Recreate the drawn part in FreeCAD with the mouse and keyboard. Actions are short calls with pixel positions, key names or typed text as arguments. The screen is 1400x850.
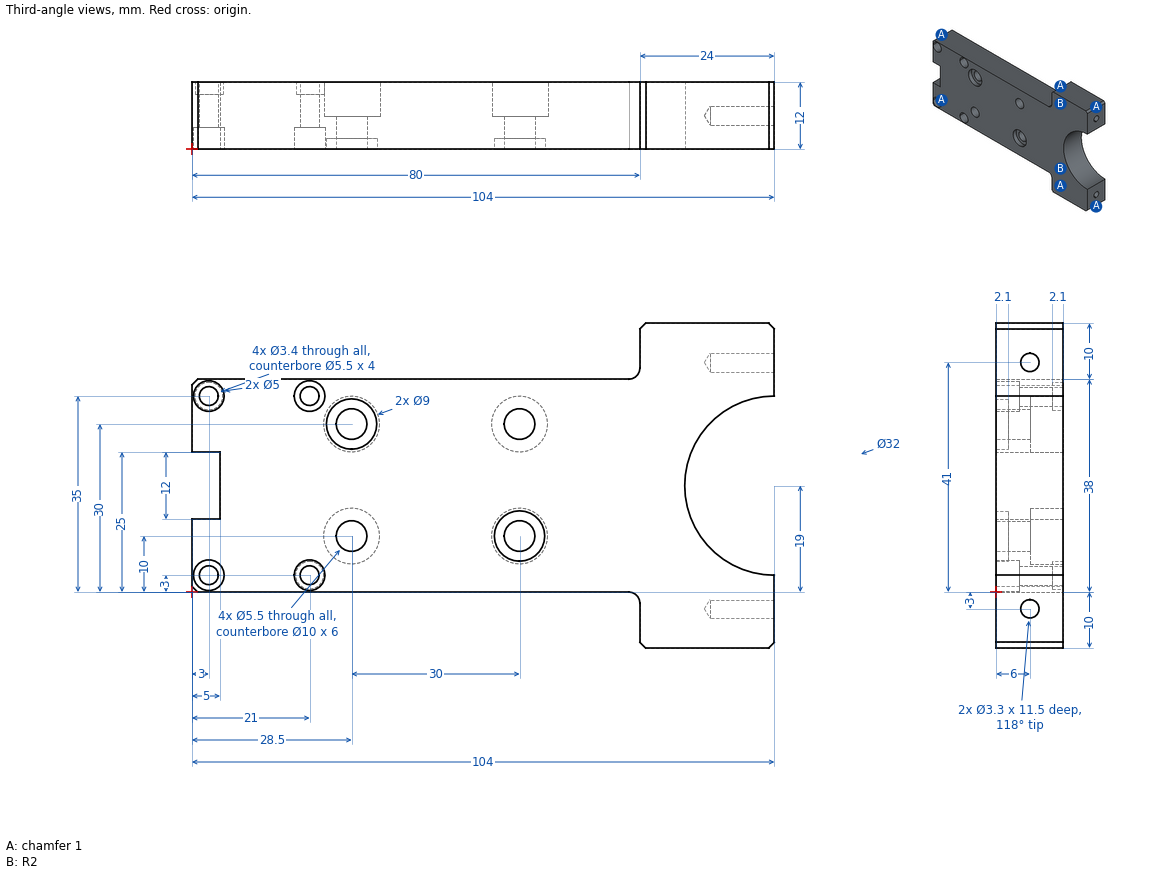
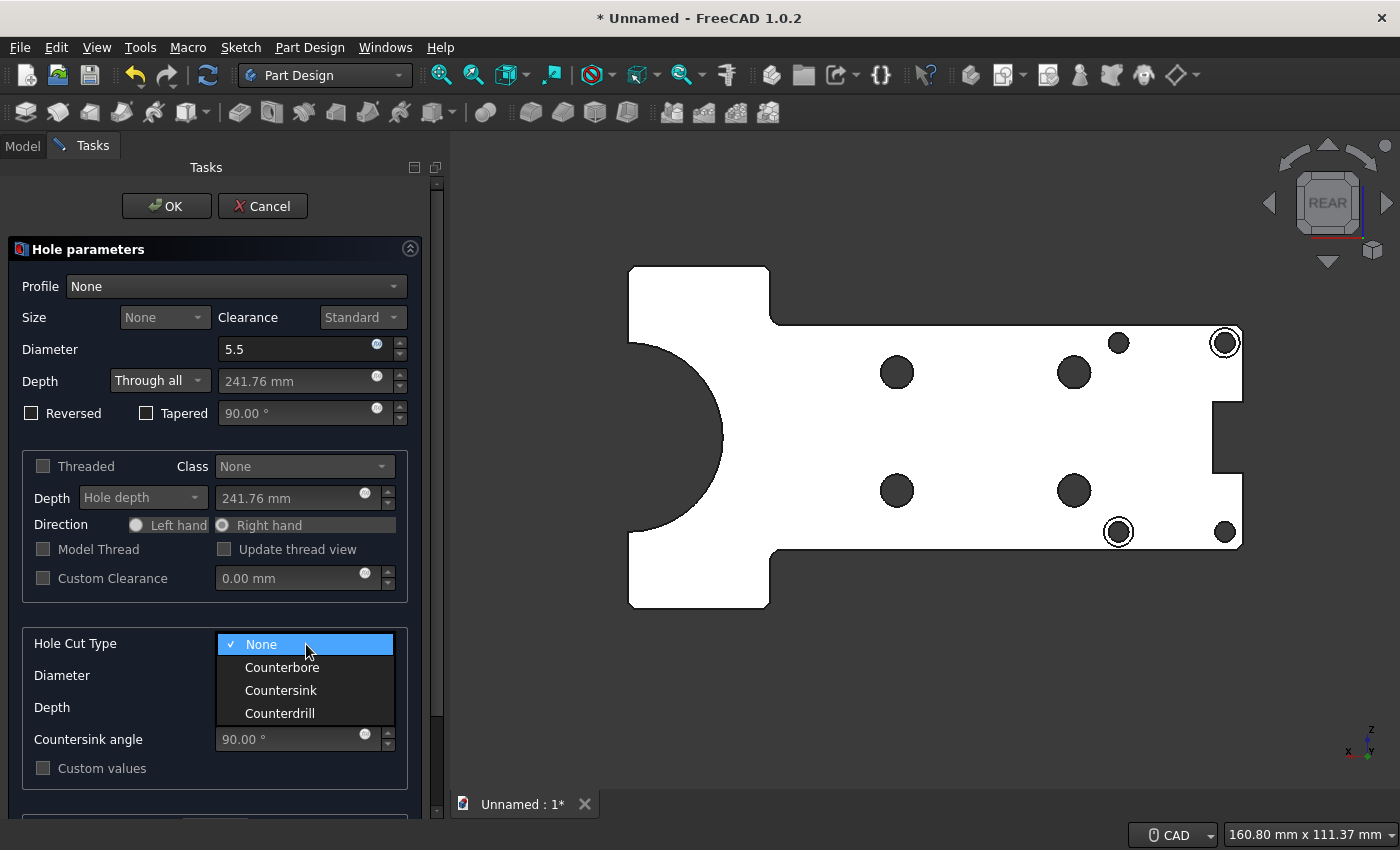
click(304, 668)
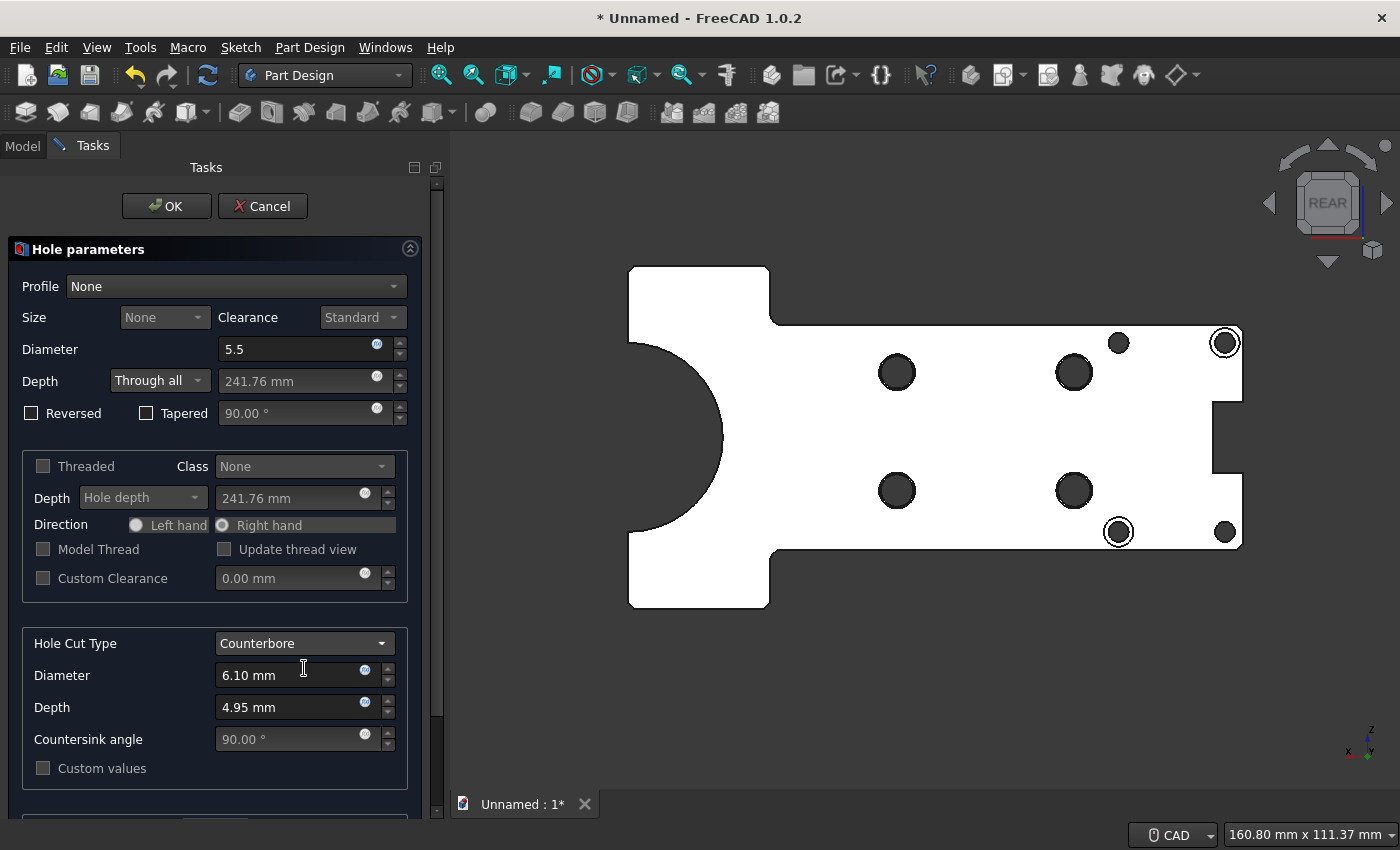
triple_click(298, 675)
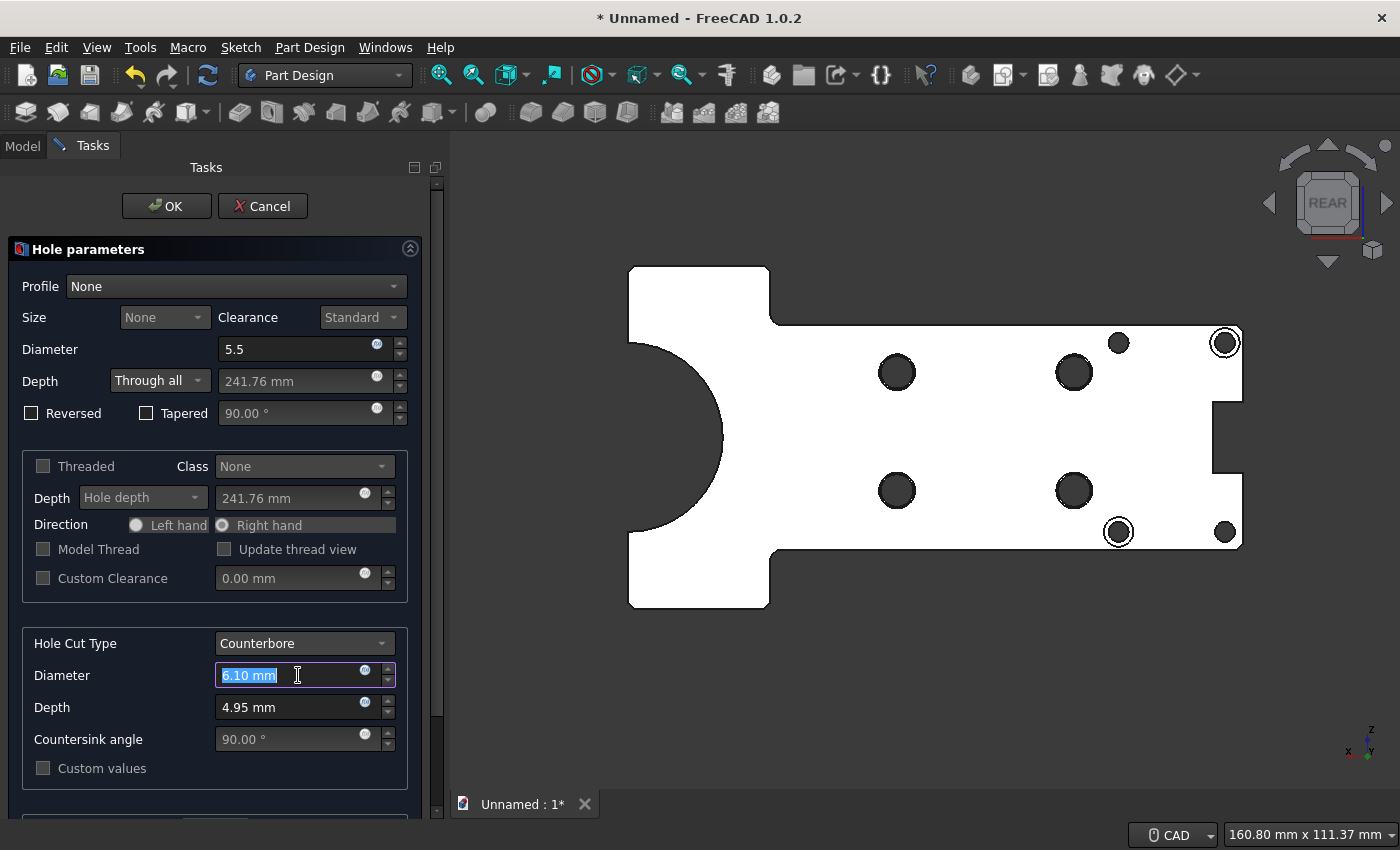
text(10)
key(Tab)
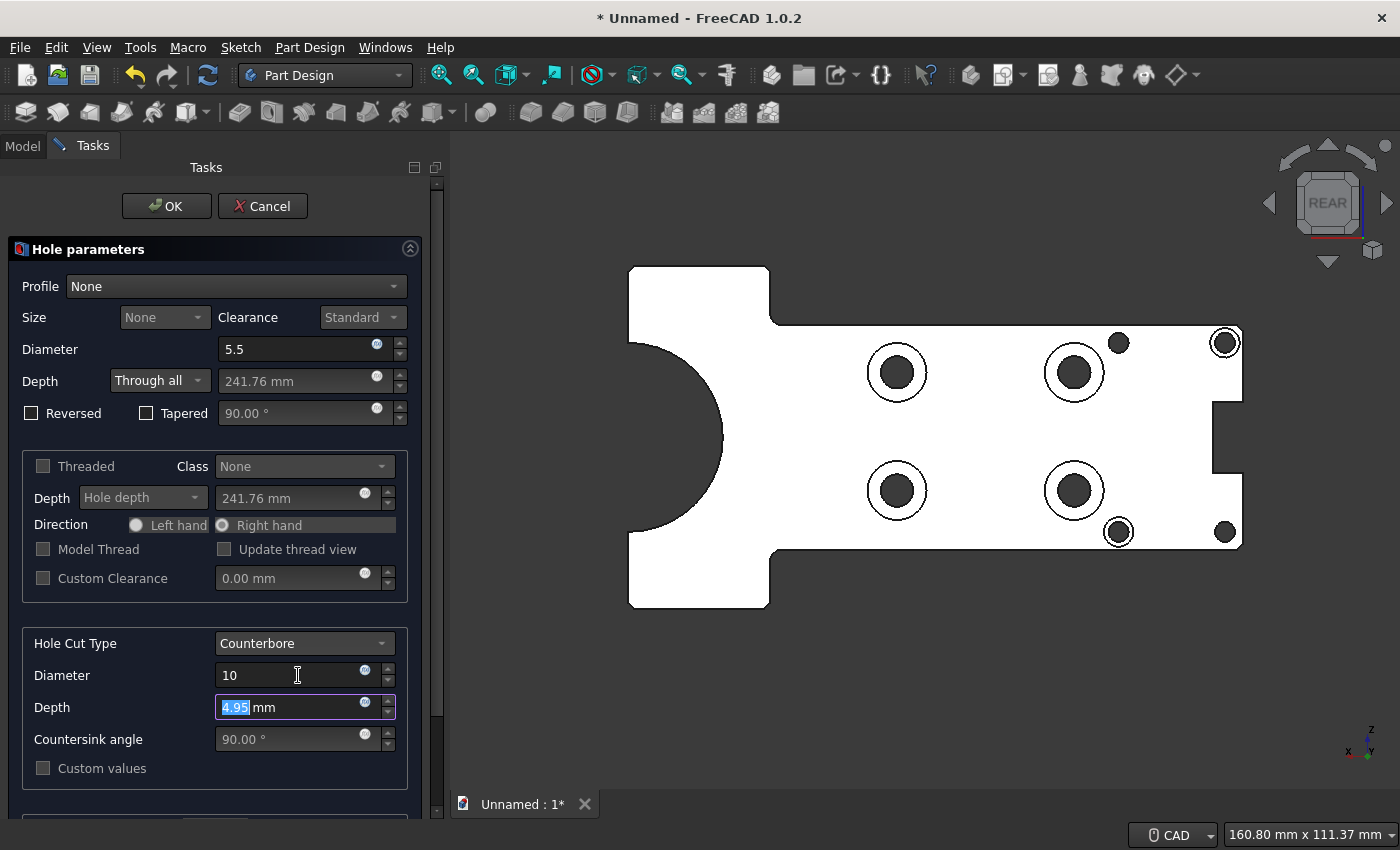
text(6)
key(Tab)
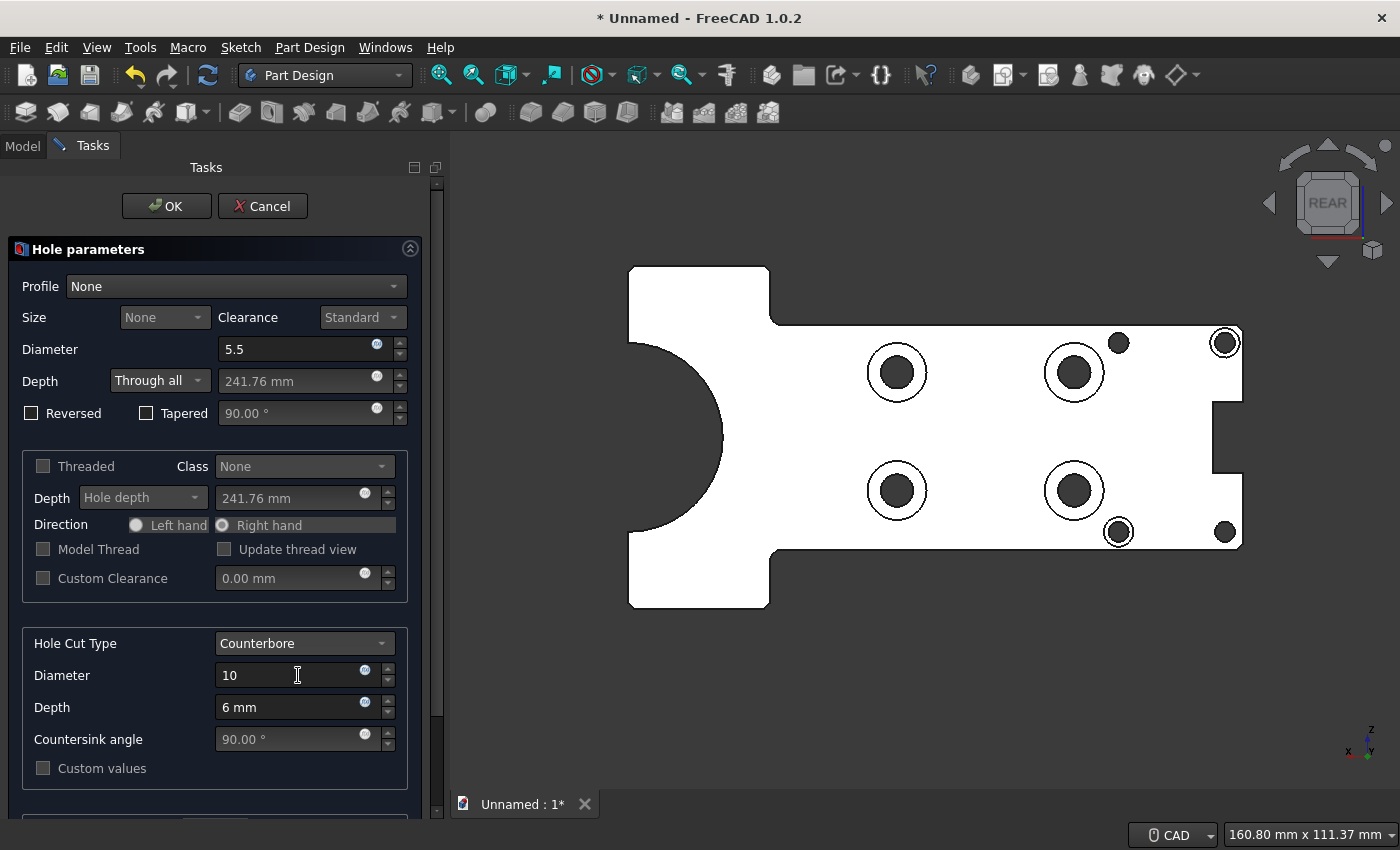
click(167, 206)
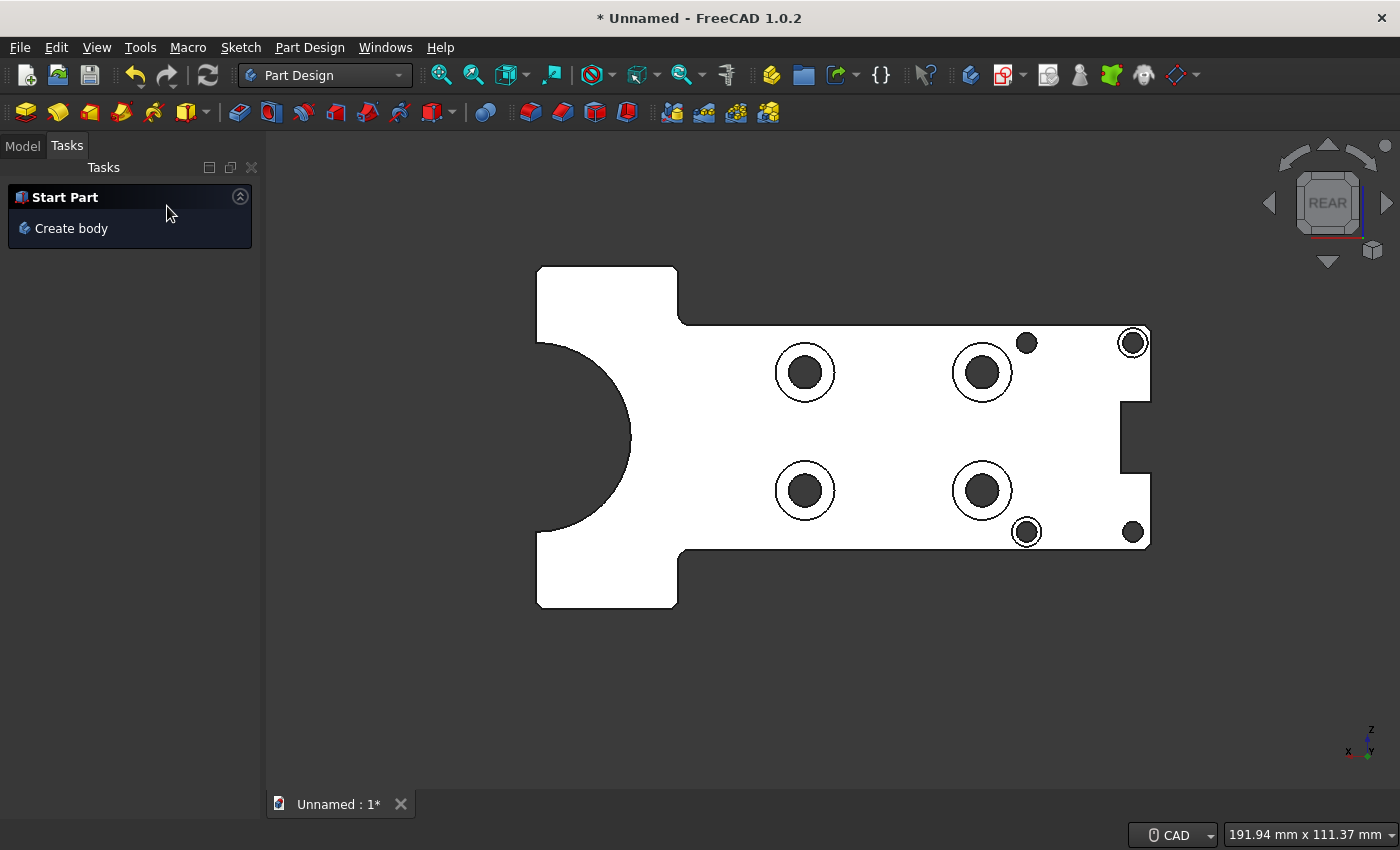
click(1004, 76)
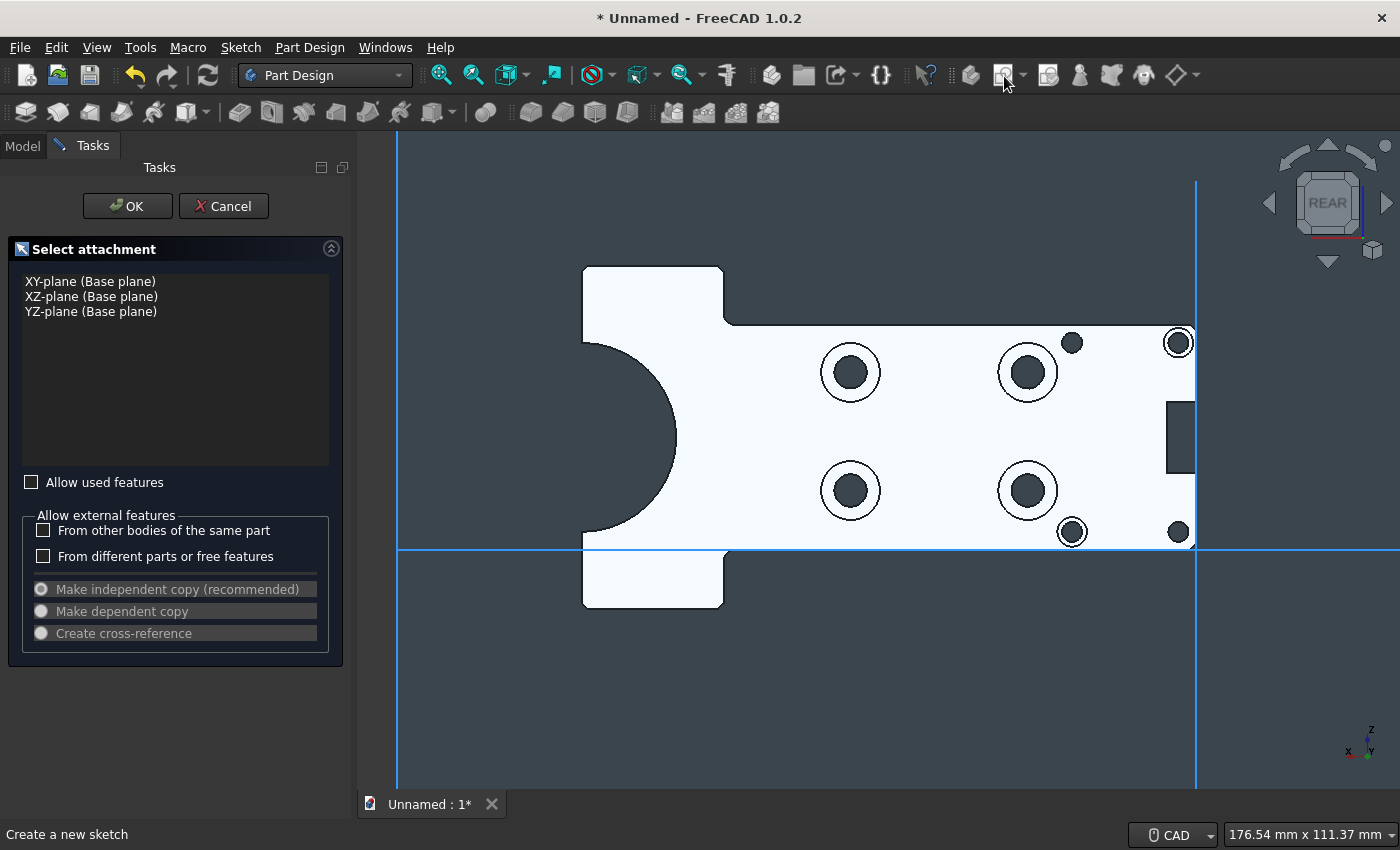
click(82, 296)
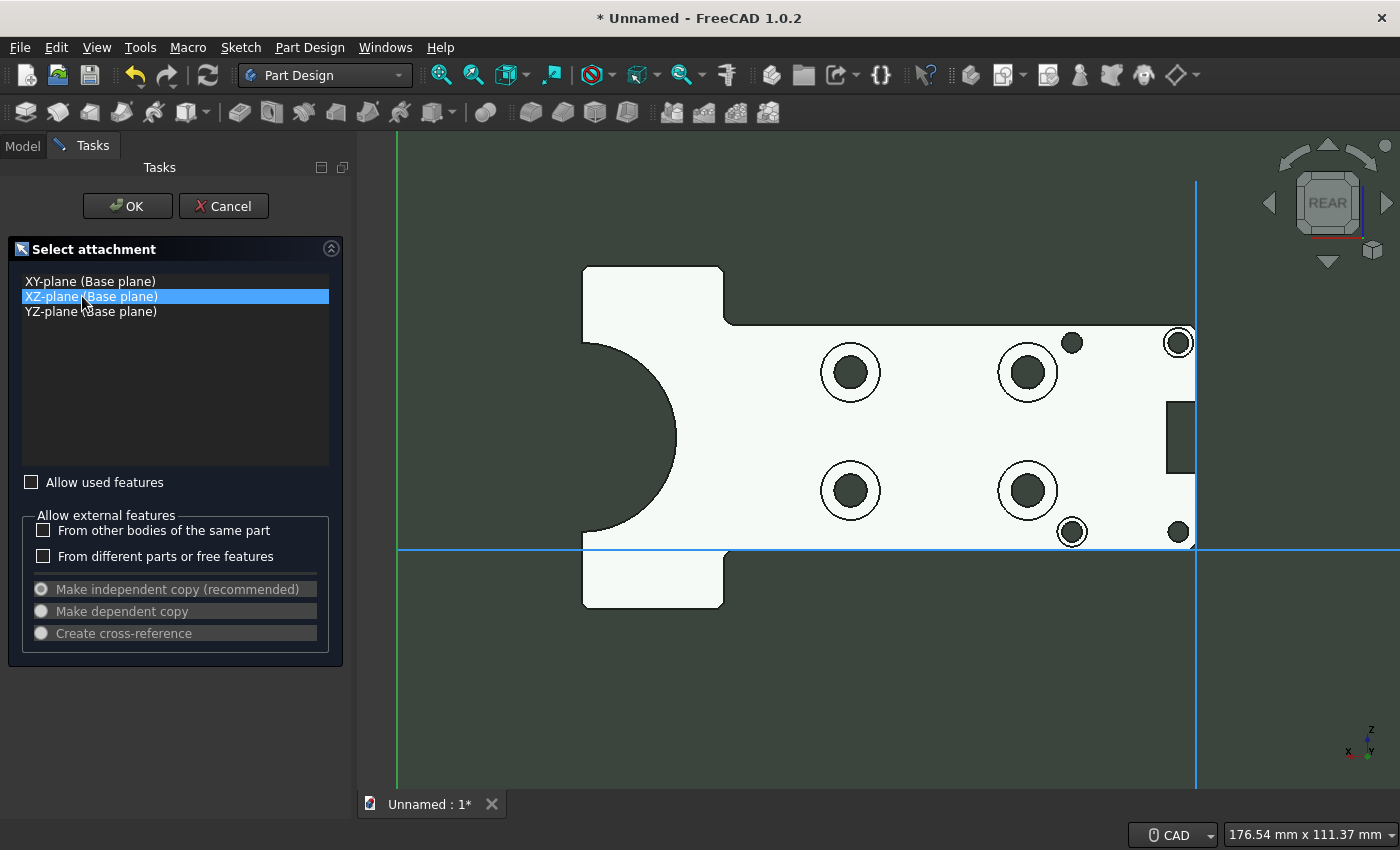
click(128, 206)